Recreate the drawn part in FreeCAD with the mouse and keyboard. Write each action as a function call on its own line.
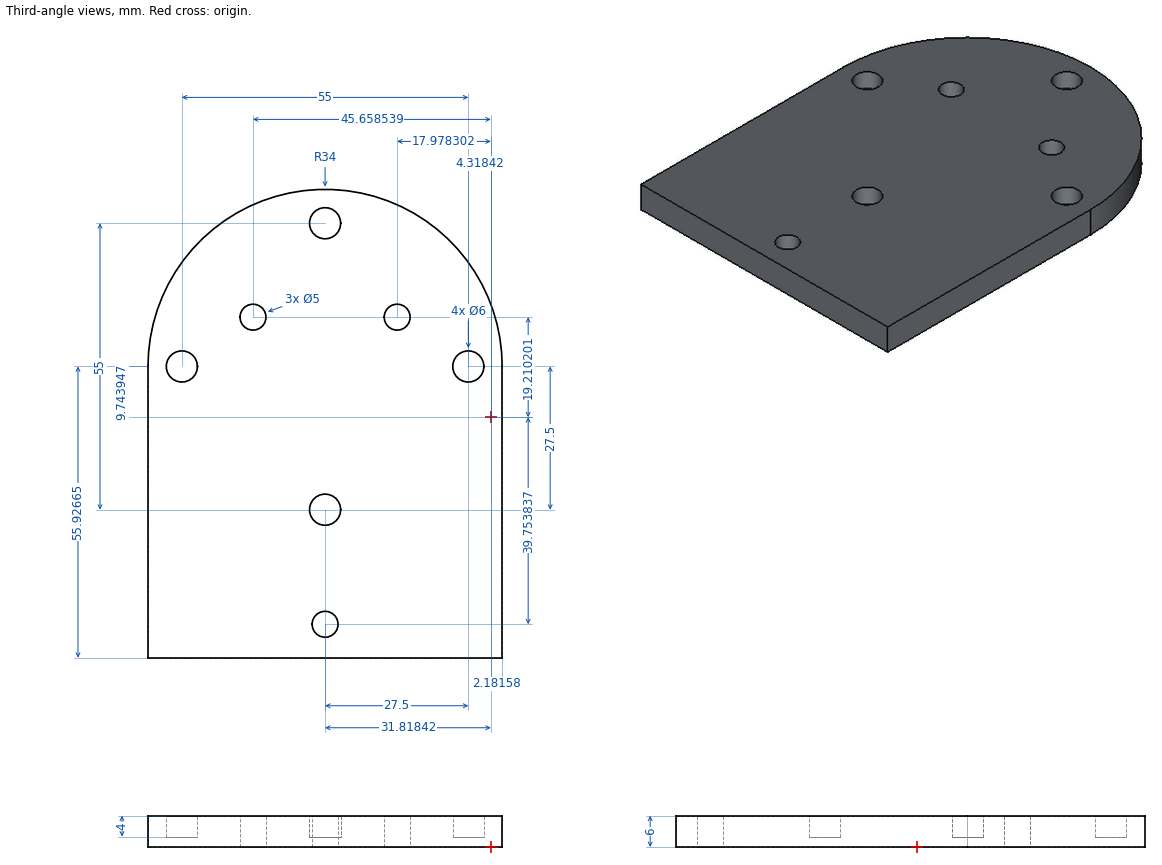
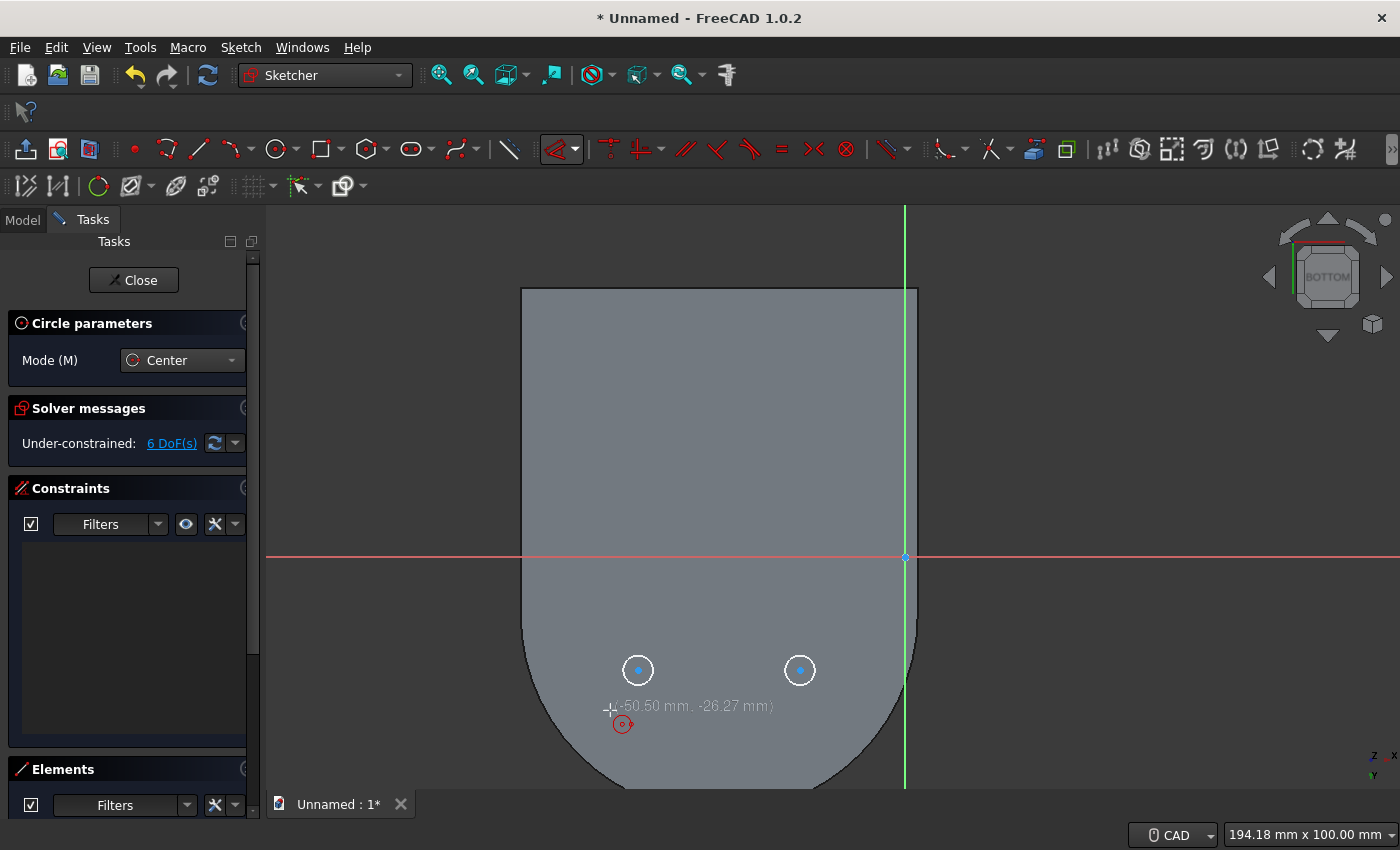
scroll(719, 325, up, 3)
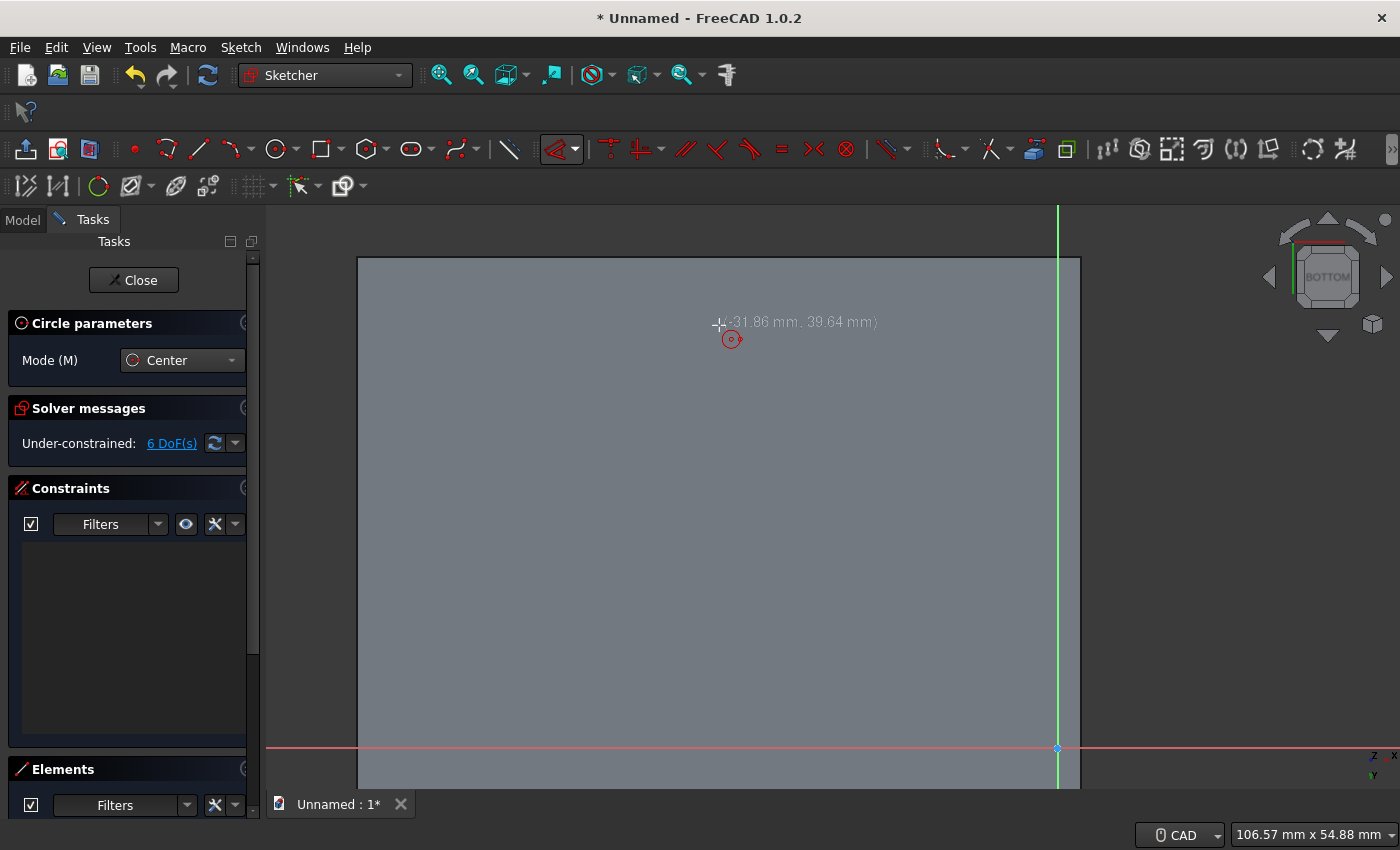
click(719, 325)
click(738, 307)
key(Escape)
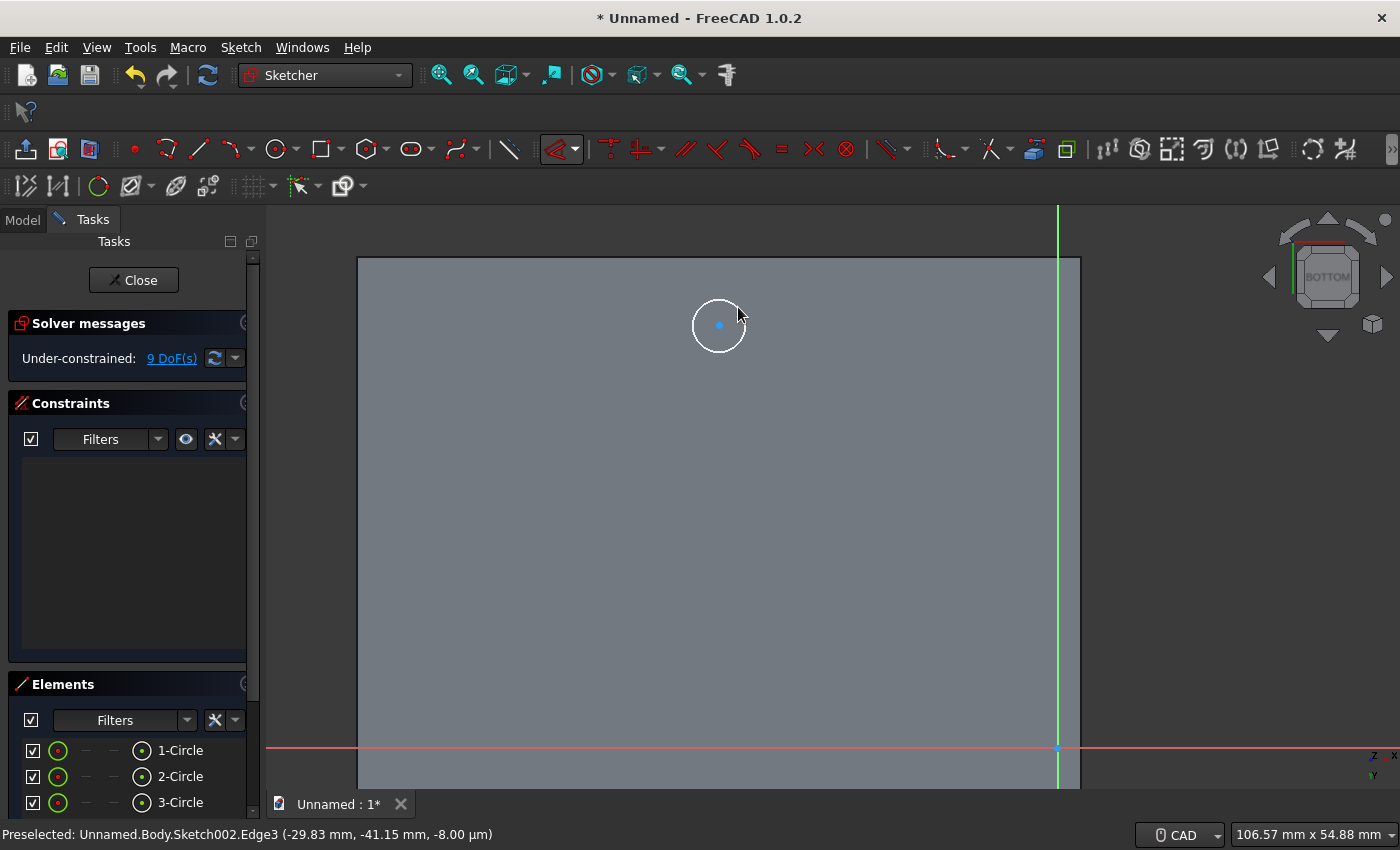
scroll(720, 324, down, 3)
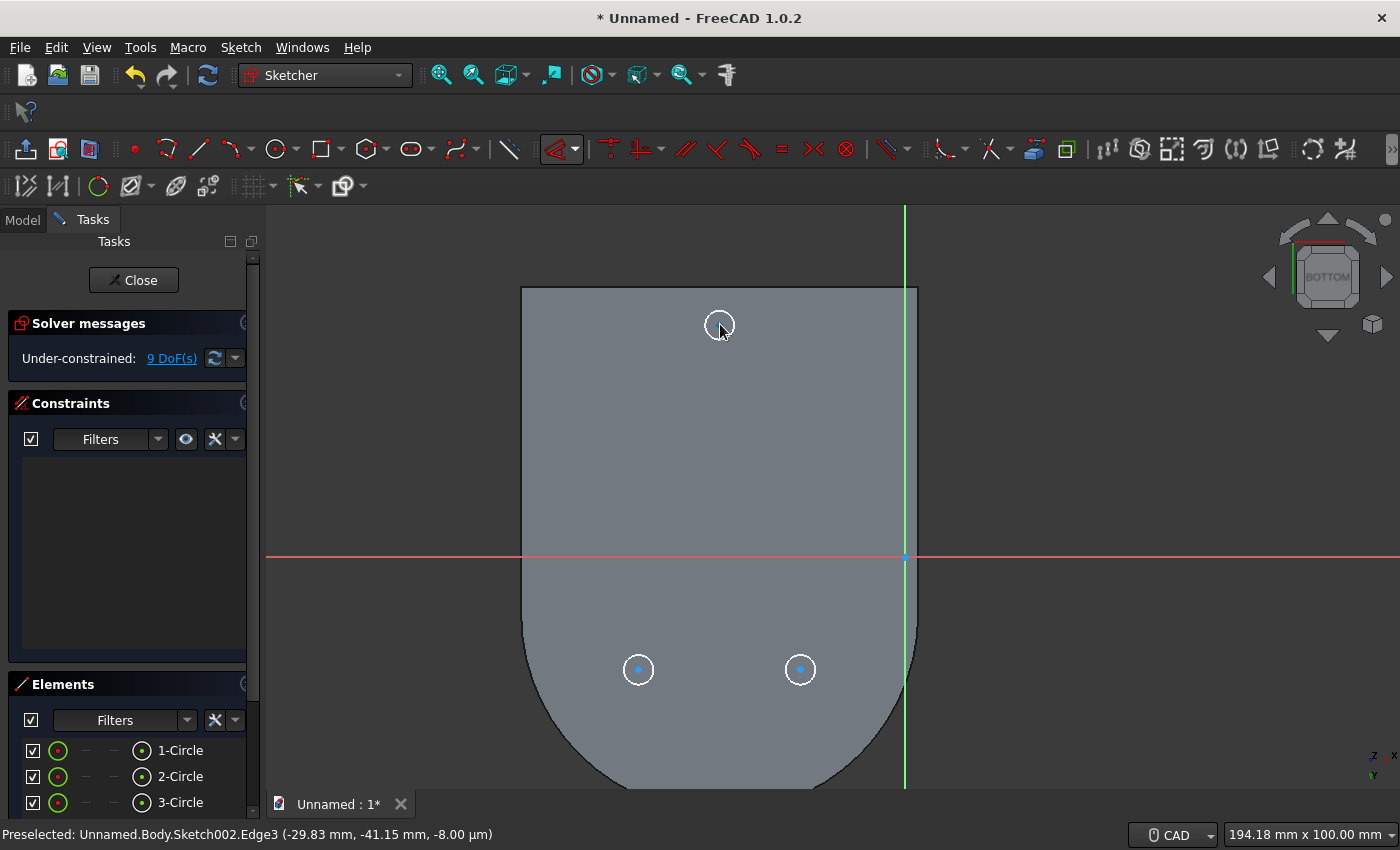
click(649, 659)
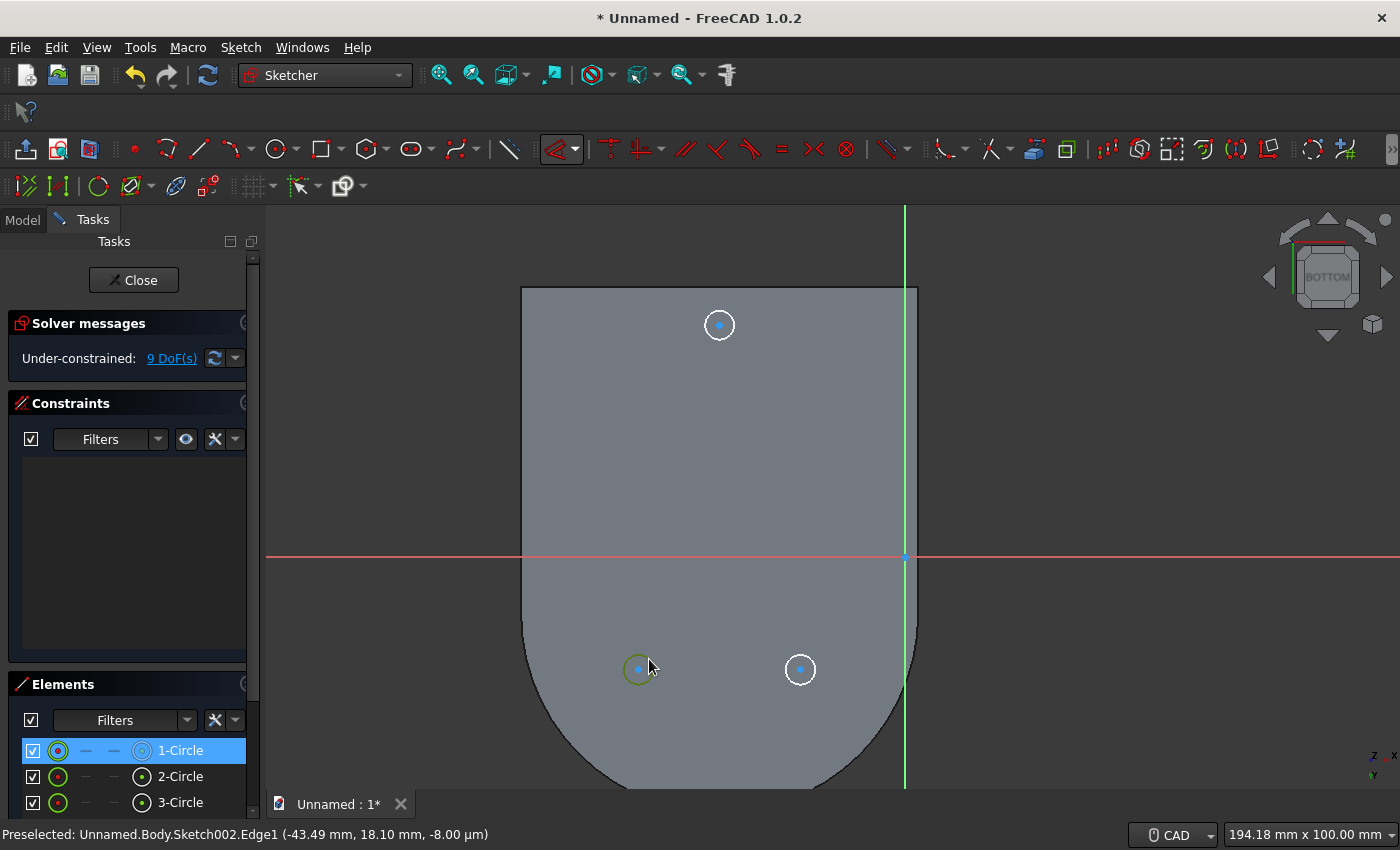
click(811, 659)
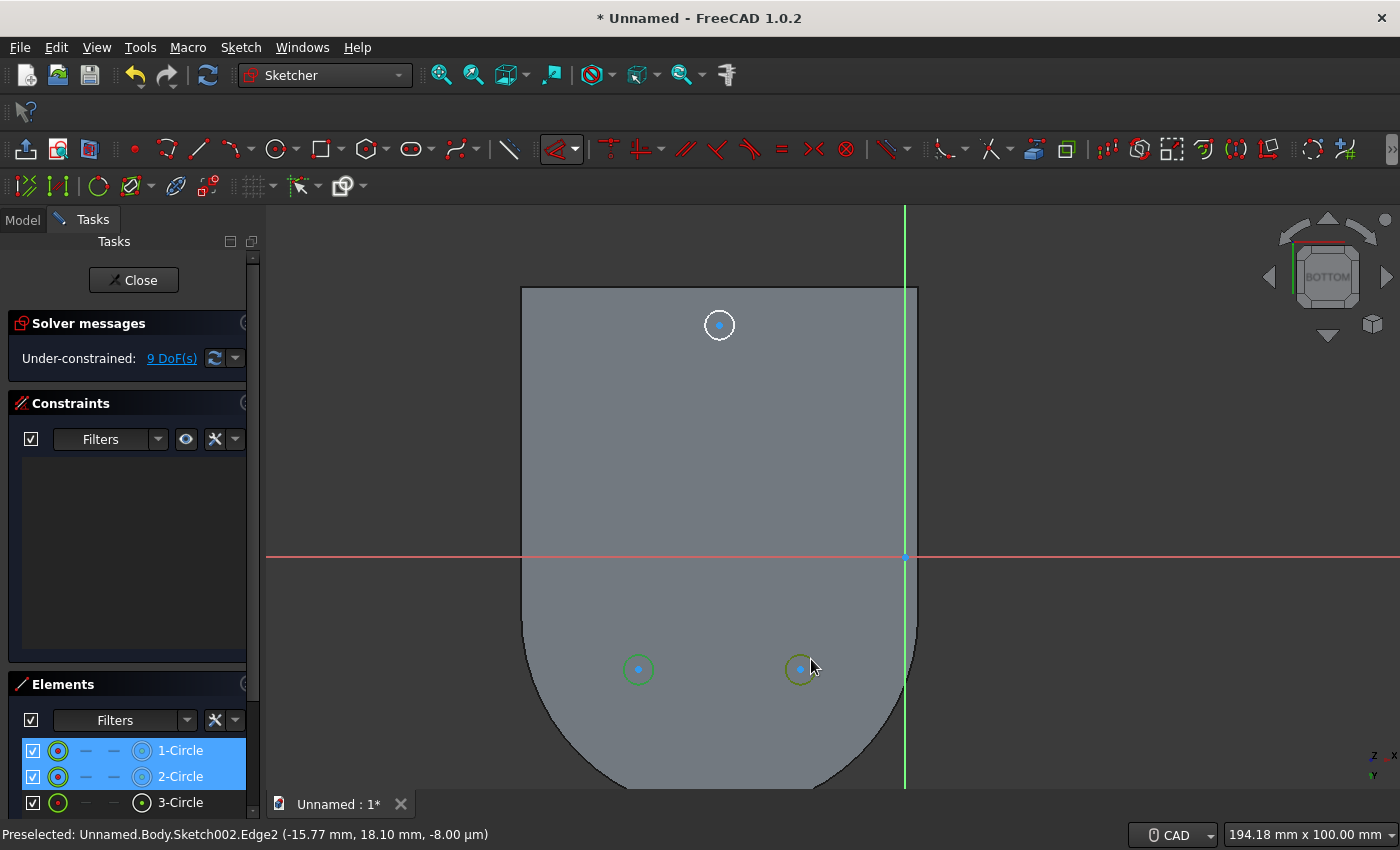
click(730, 315)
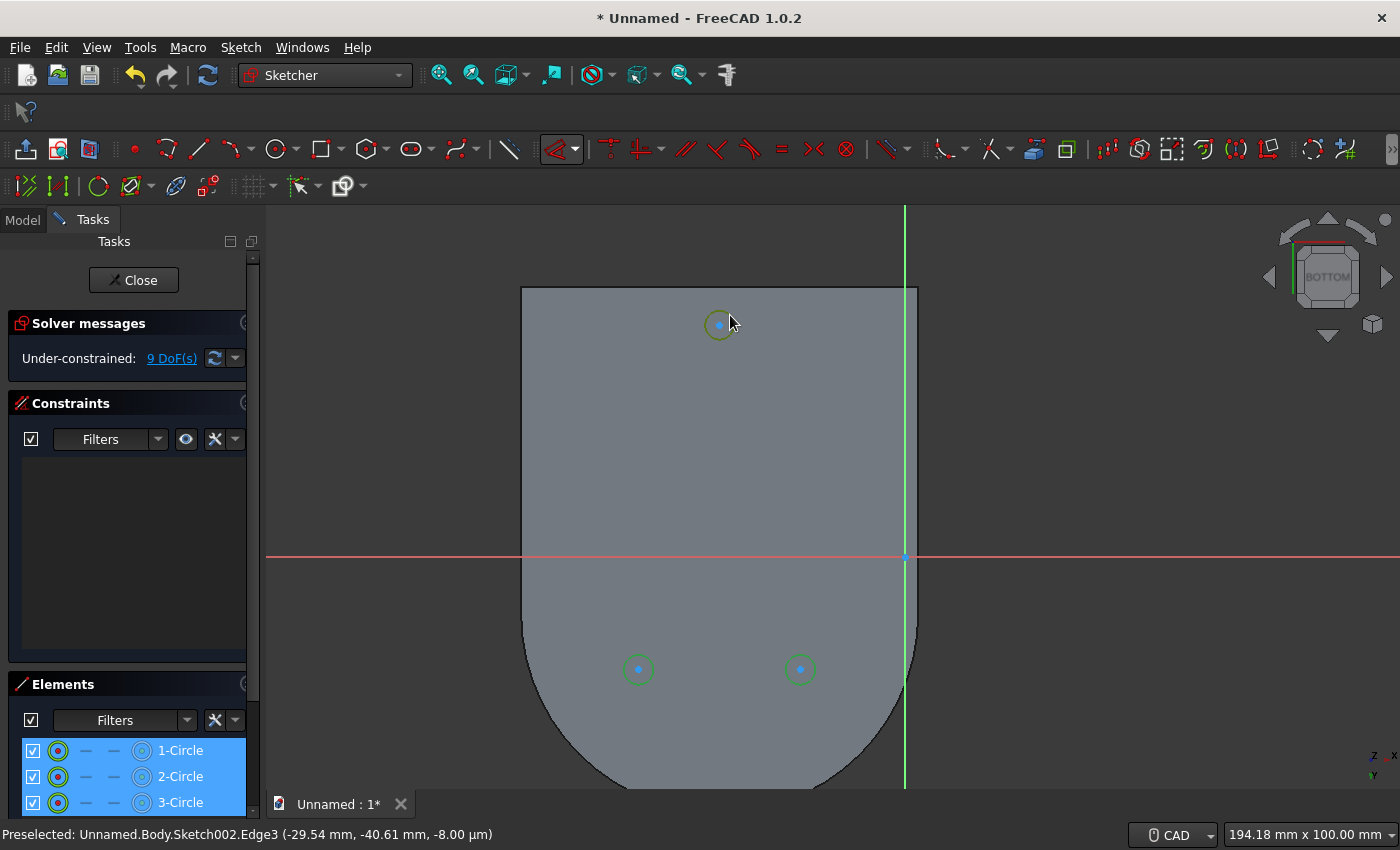
key(e)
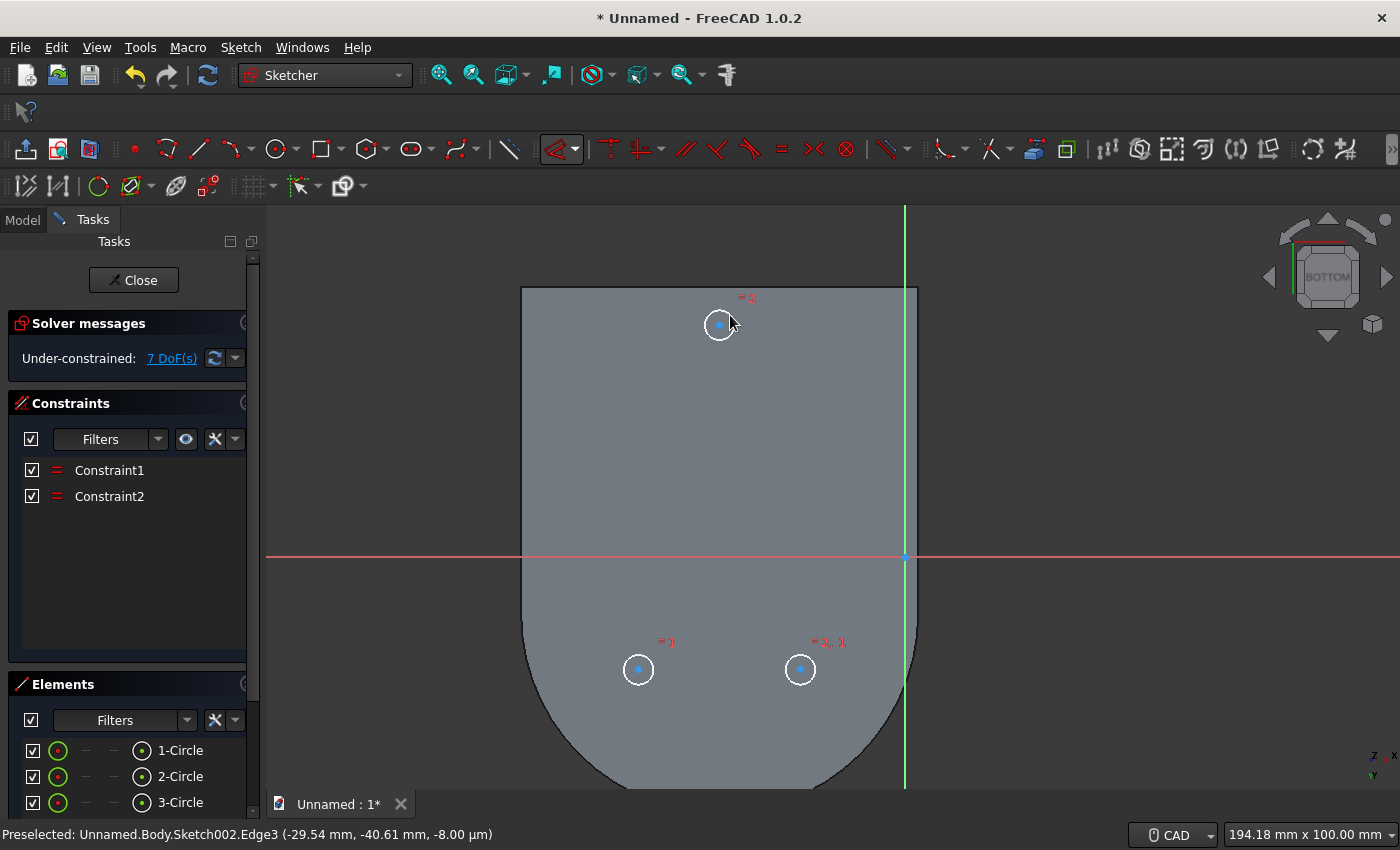
click(639, 670)